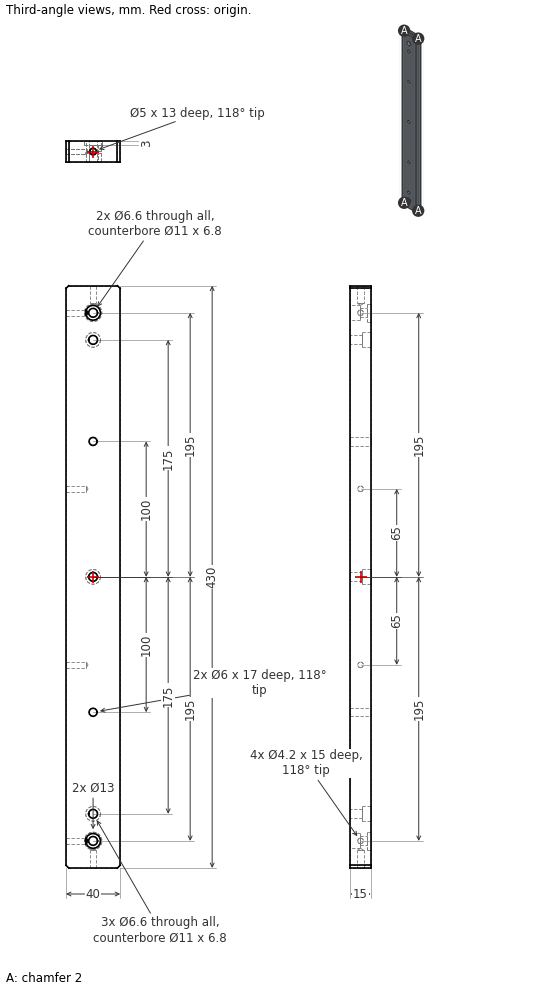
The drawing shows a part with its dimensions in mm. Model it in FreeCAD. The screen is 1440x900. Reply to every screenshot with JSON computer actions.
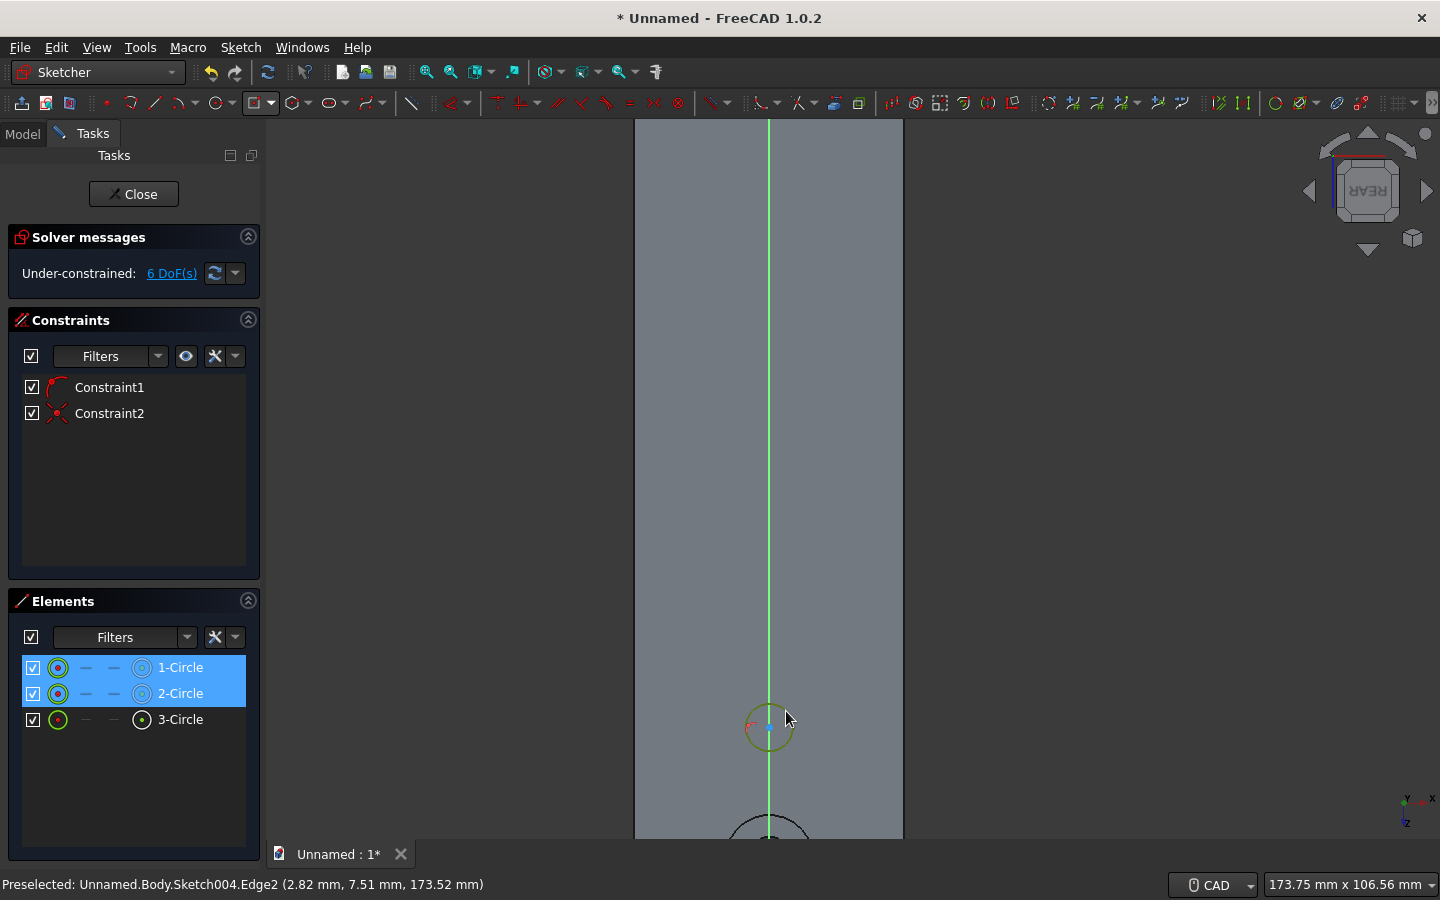
{"action": "scroll", "coordinate": [788, 716], "scroll_direction": "down", "scroll_amount": 8}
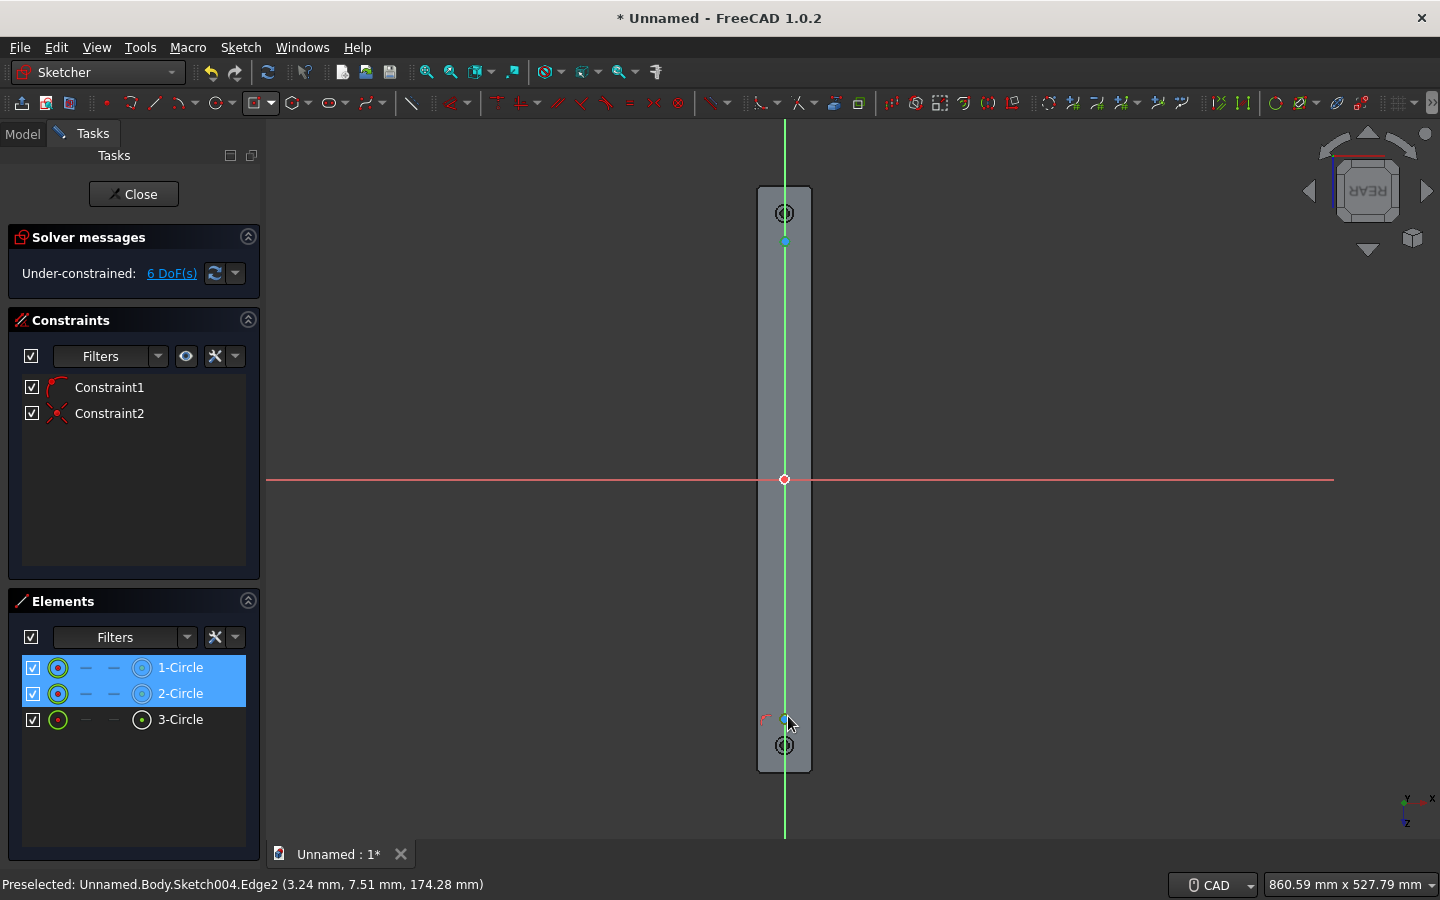
{"action": "scroll", "coordinate": [788, 476], "scroll_direction": "up", "scroll_amount": 8}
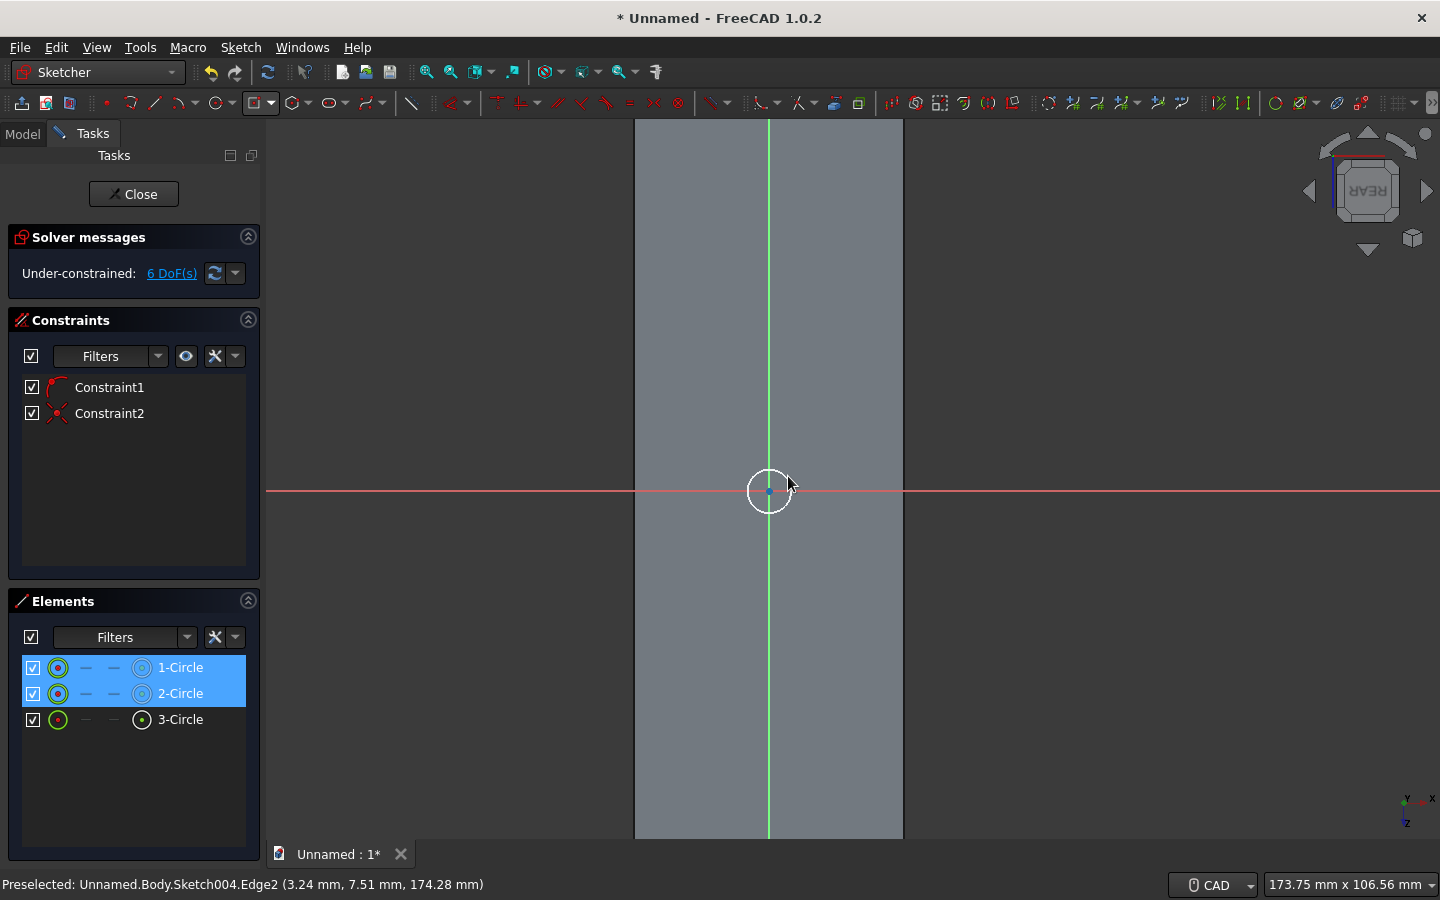
{"action": "left_click", "coordinate": [785, 476]}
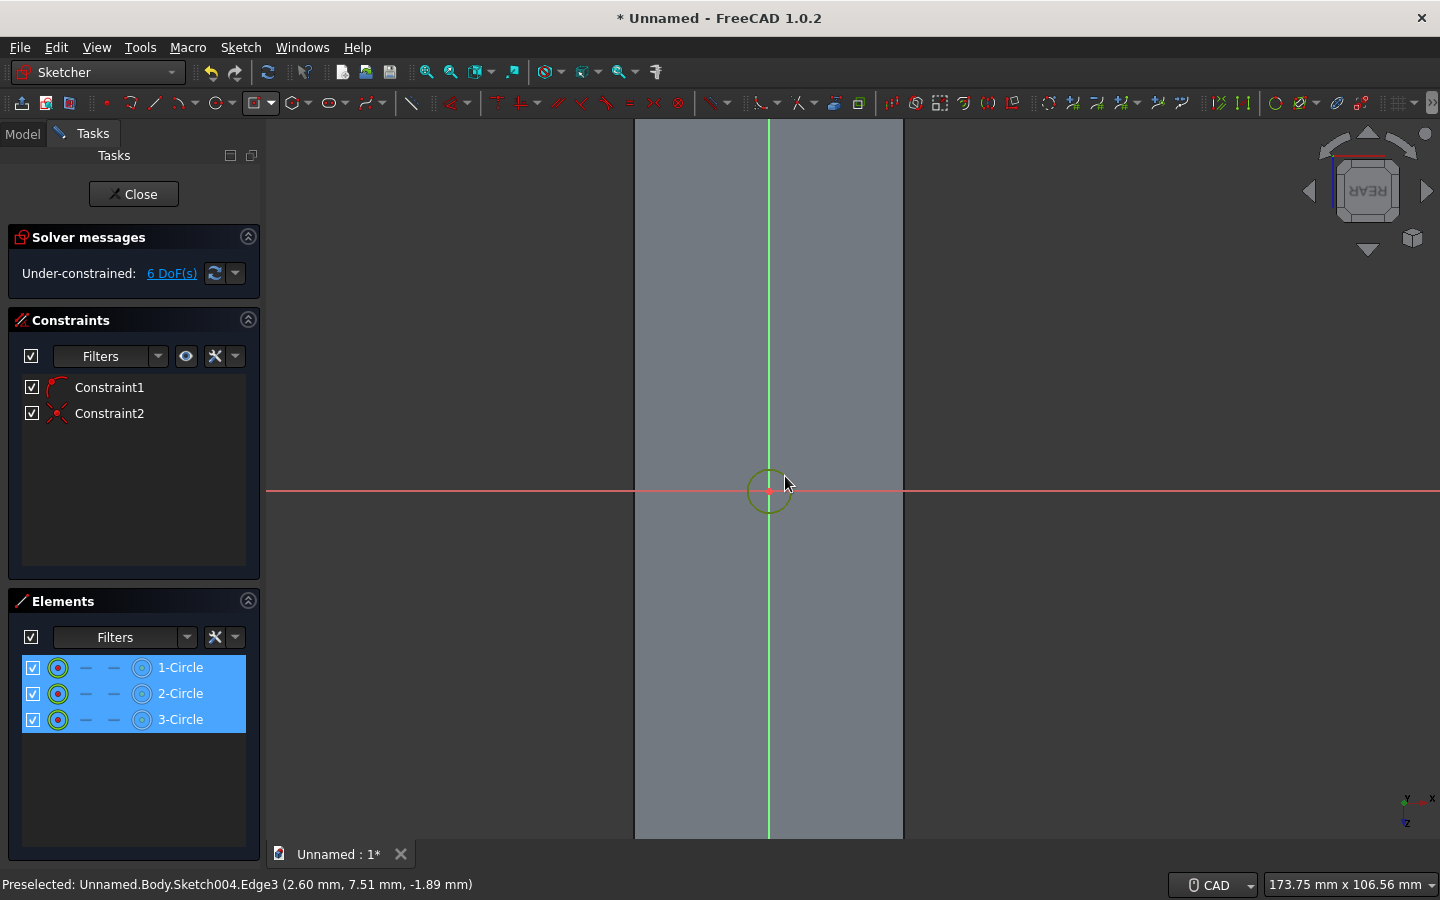
{"action": "key", "text": "e"}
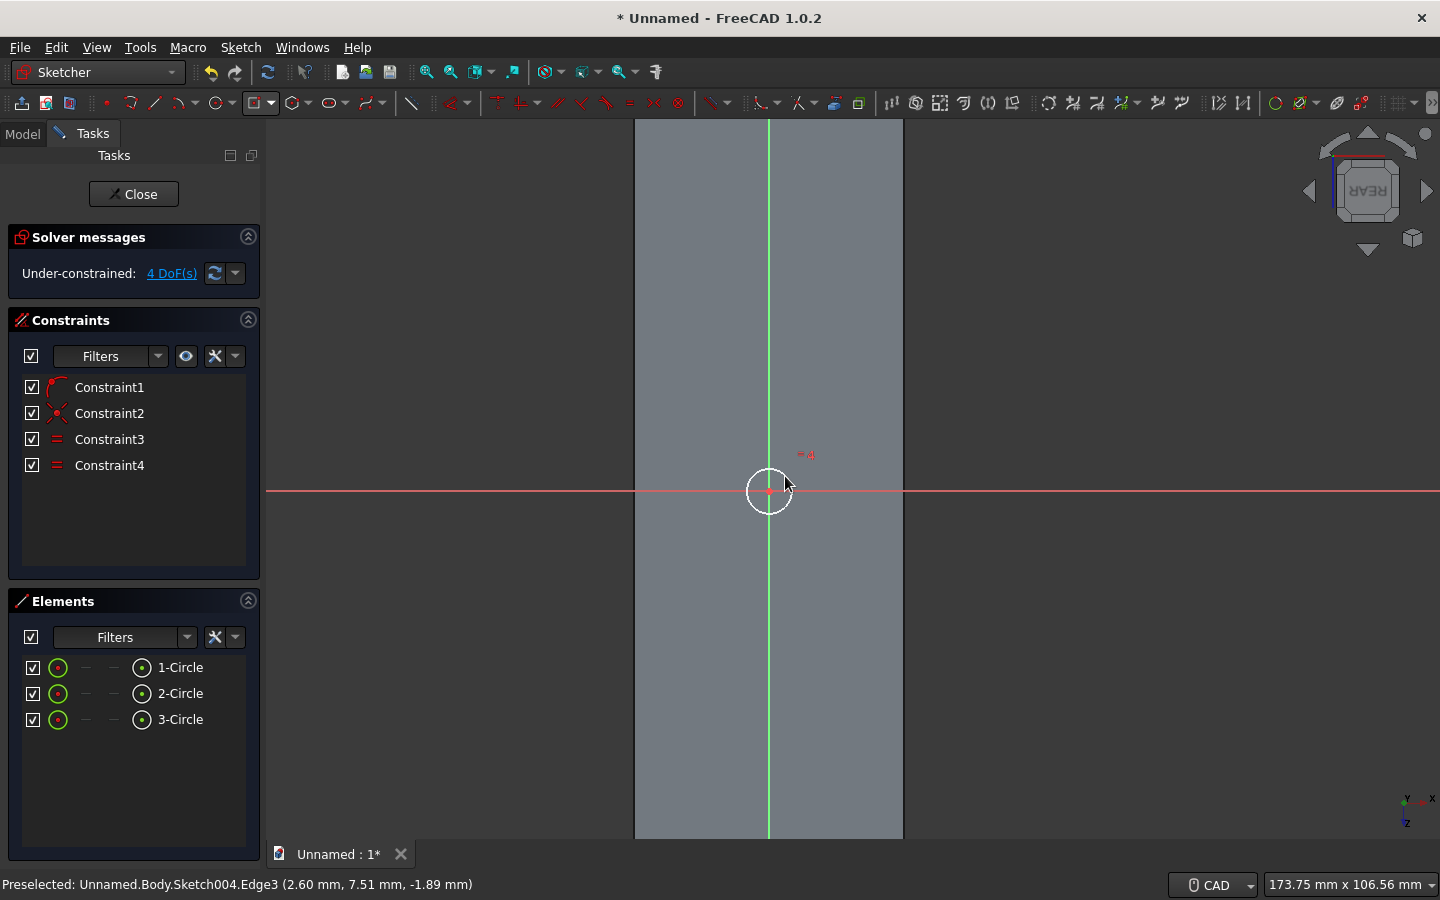
{"action": "scroll", "coordinate": [788, 476], "scroll_direction": "down", "scroll_amount": 8}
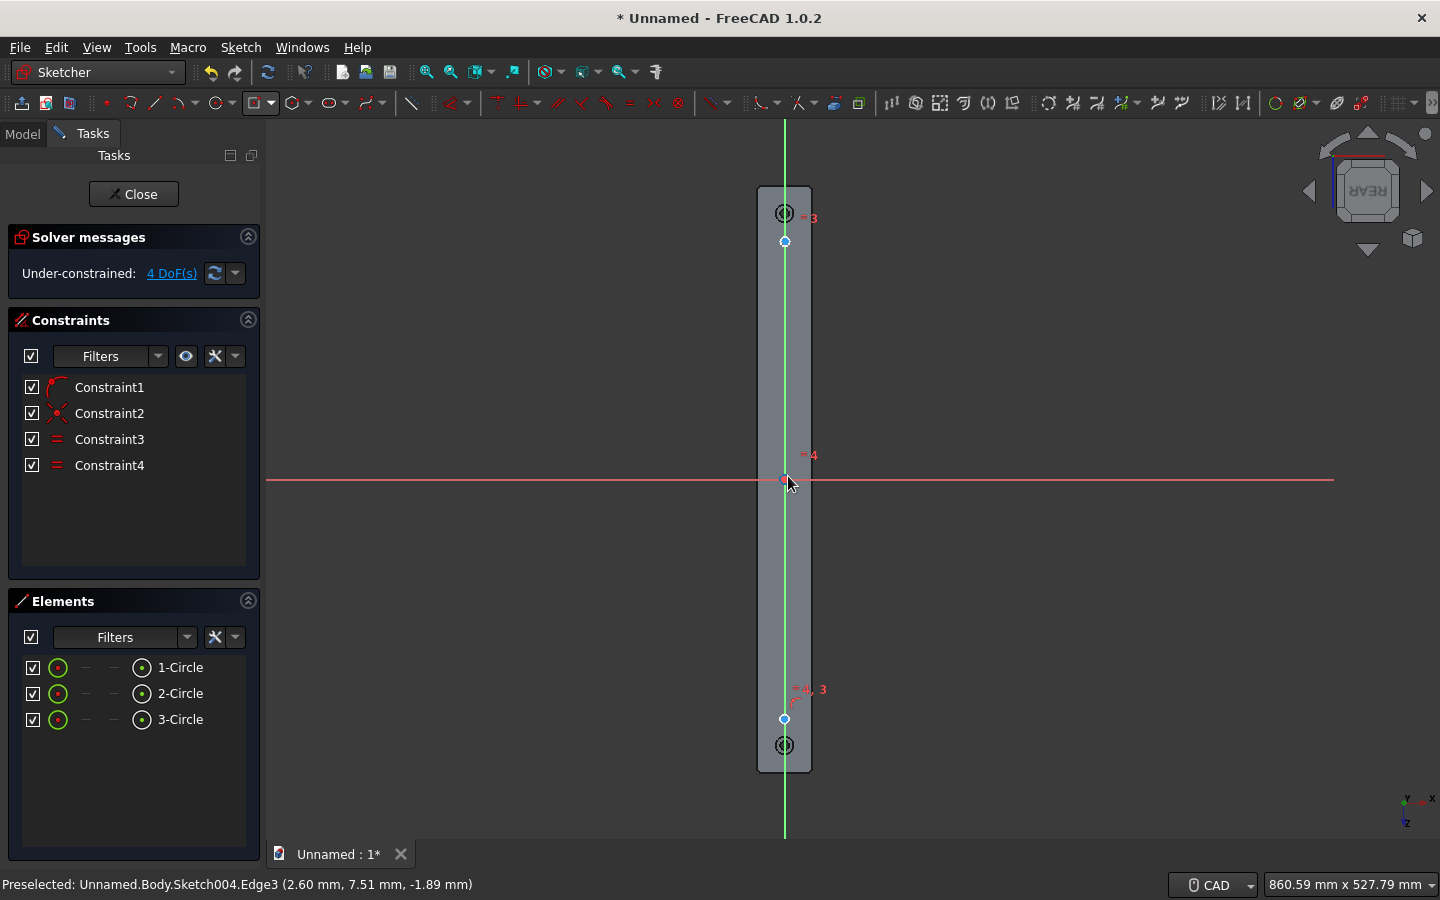
{"action": "left_click", "coordinate": [785, 242]}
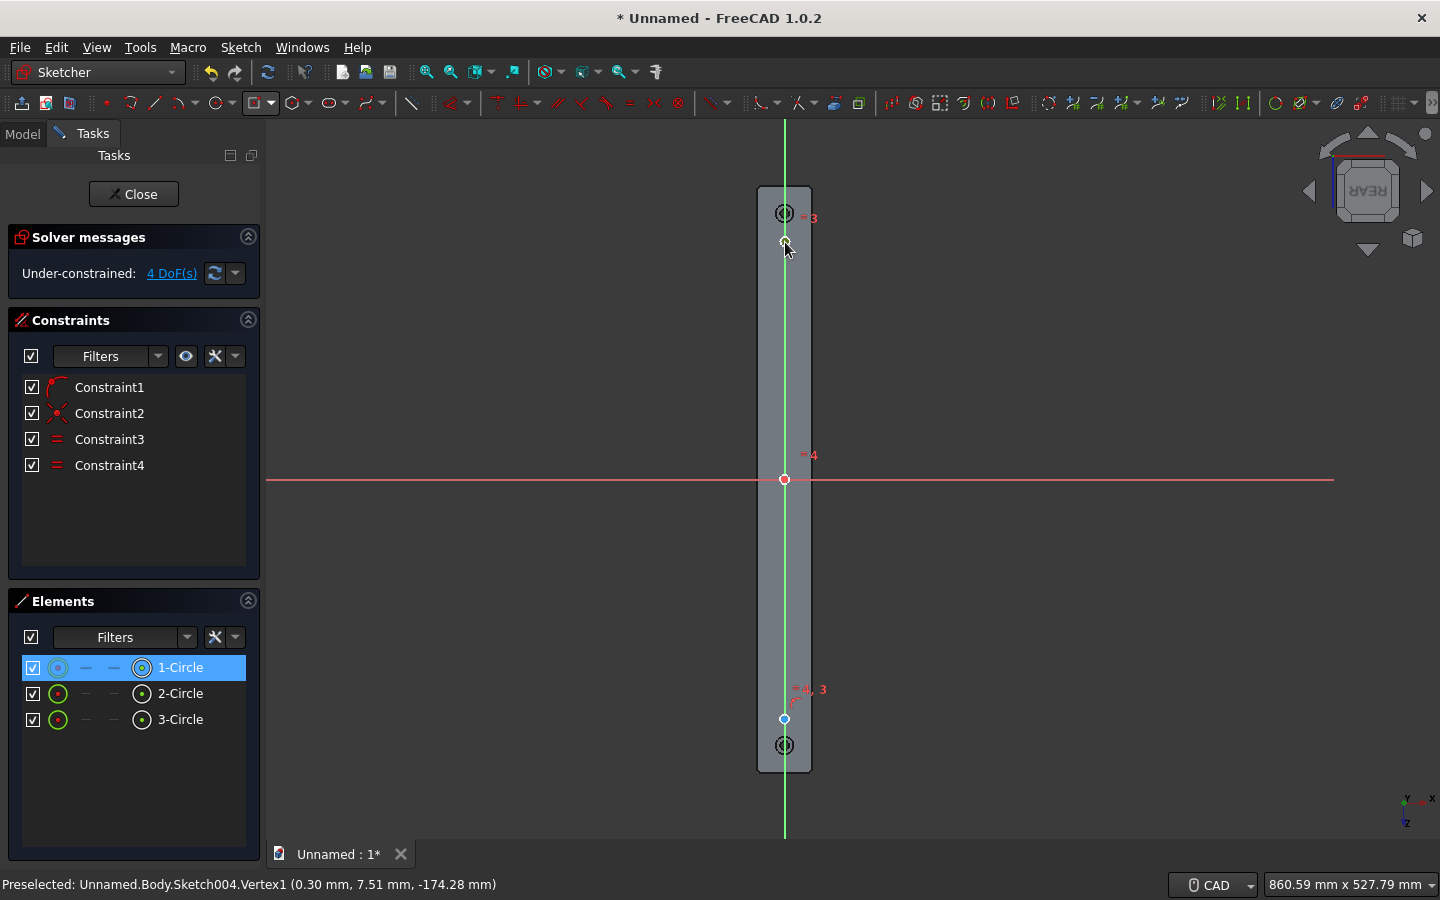
{"action": "left_click", "coordinate": [785, 764]}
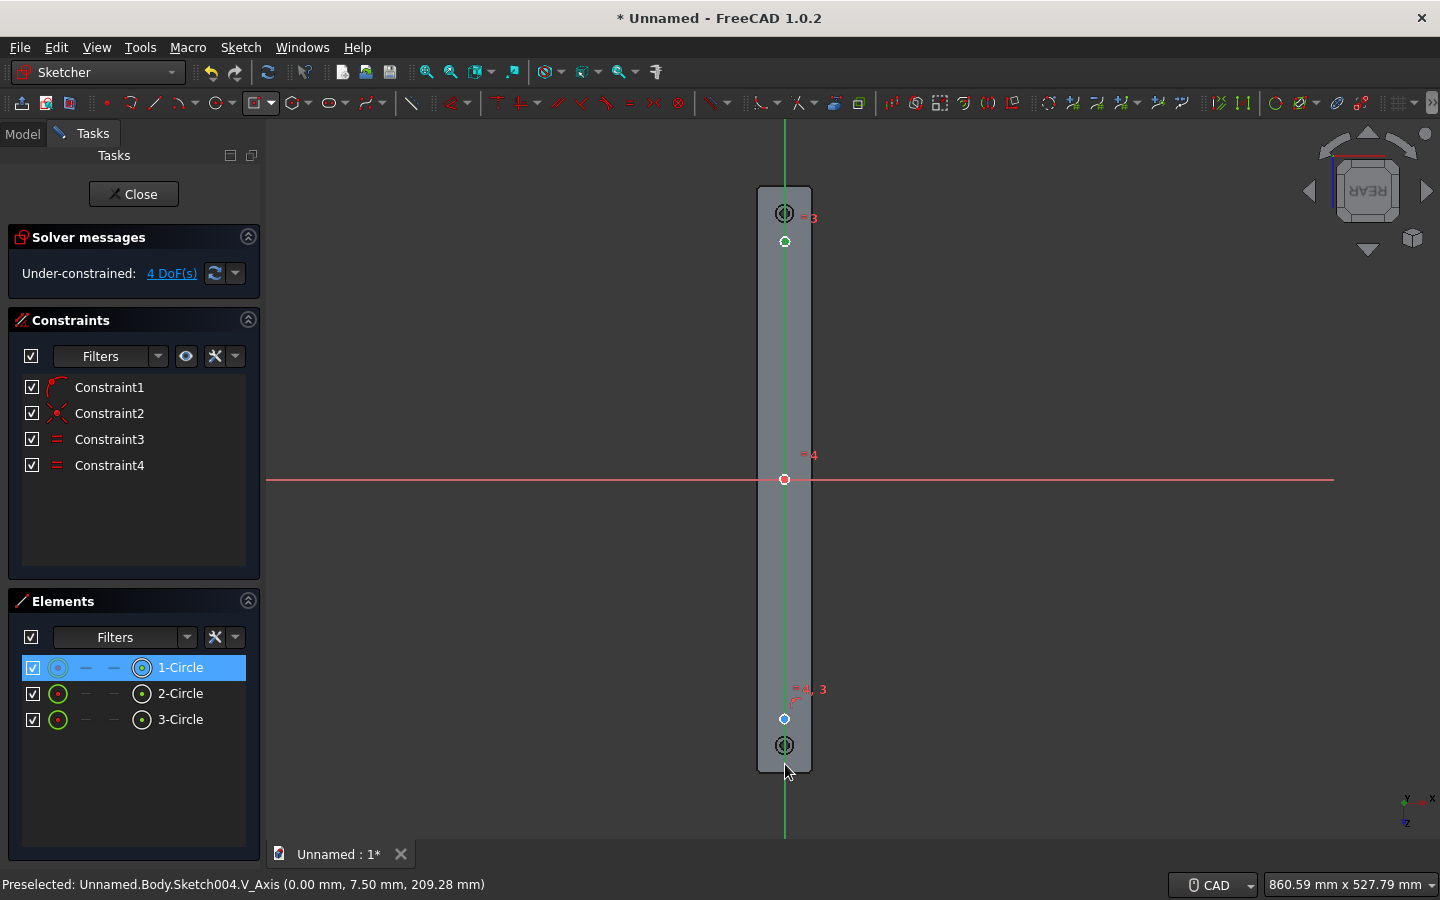
{"action": "left_click", "coordinate": [498, 104]}